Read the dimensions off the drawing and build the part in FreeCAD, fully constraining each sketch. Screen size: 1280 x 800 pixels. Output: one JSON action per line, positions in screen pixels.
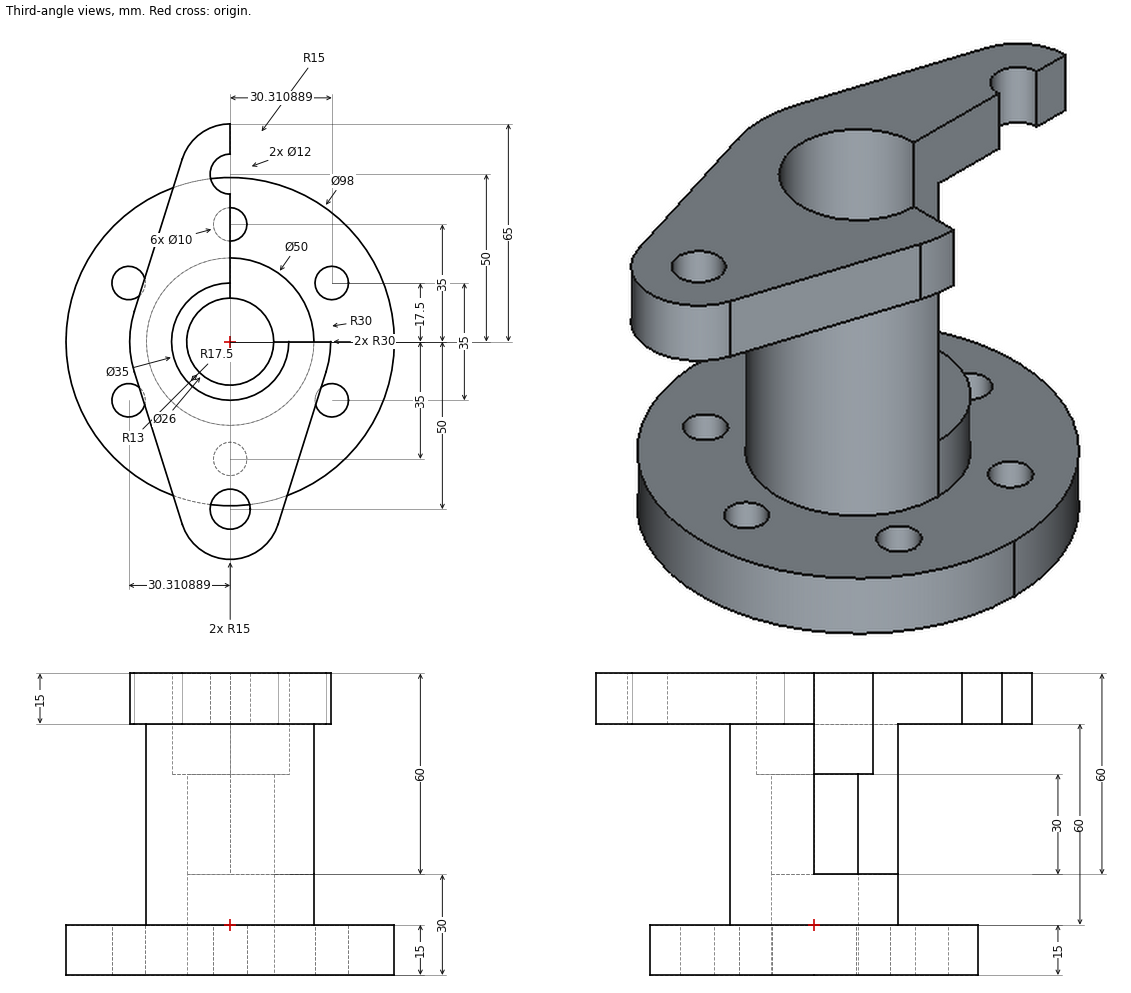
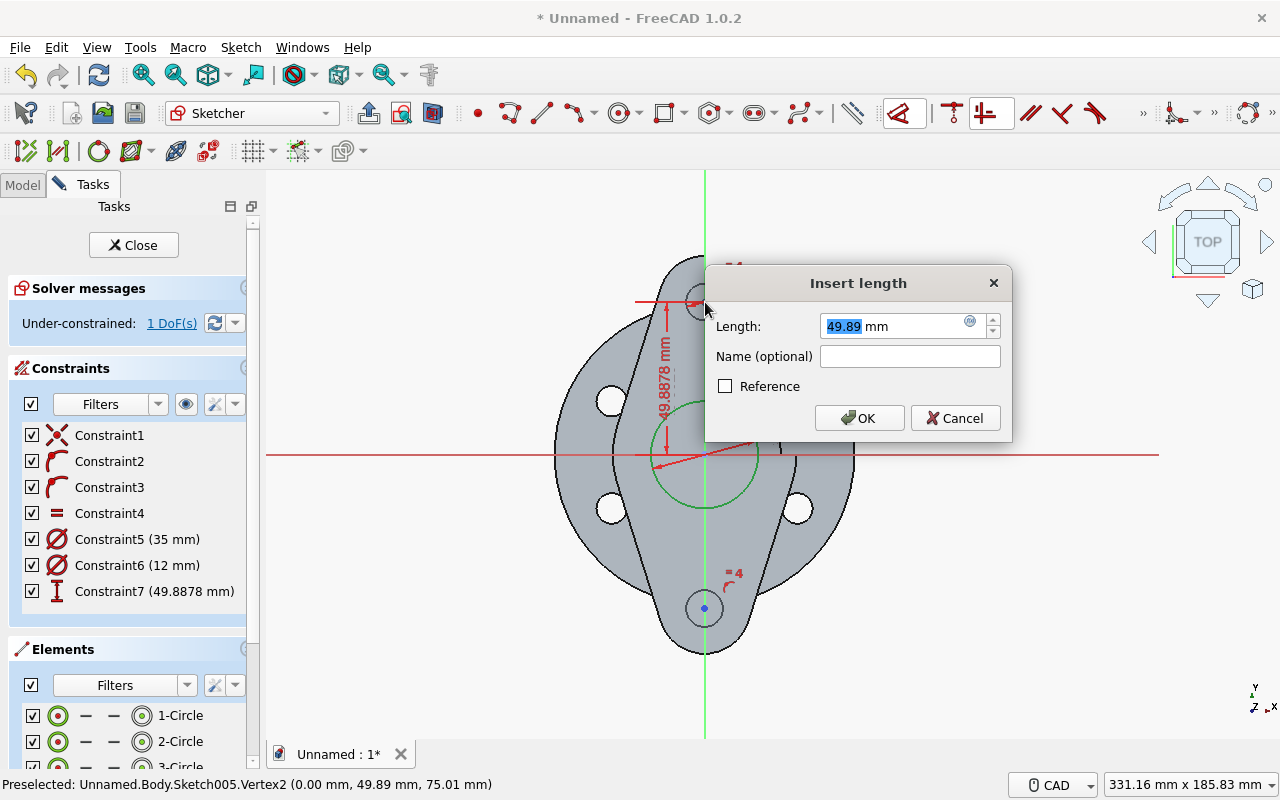
{"action": "type", "text": "50"}
{"action": "key", "text": "Return"}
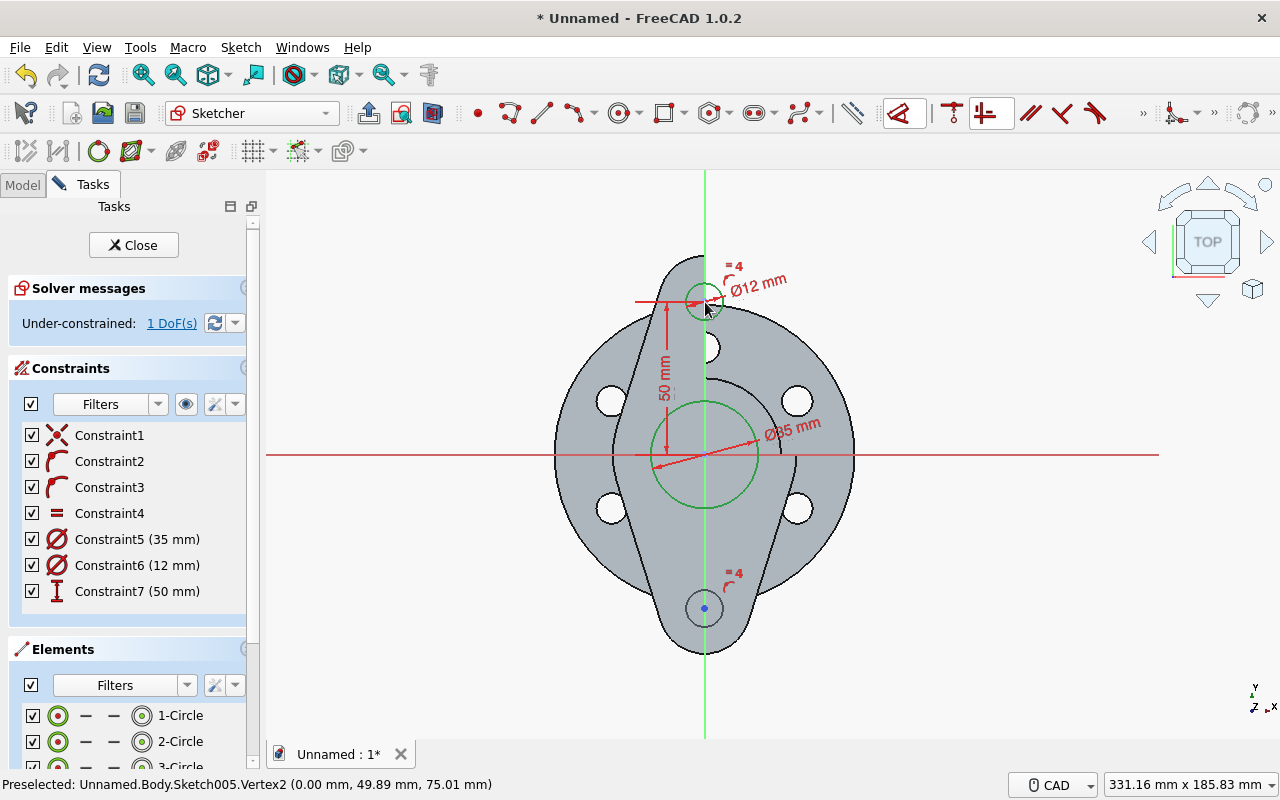
{"action": "left_click", "coordinate": [705, 609]}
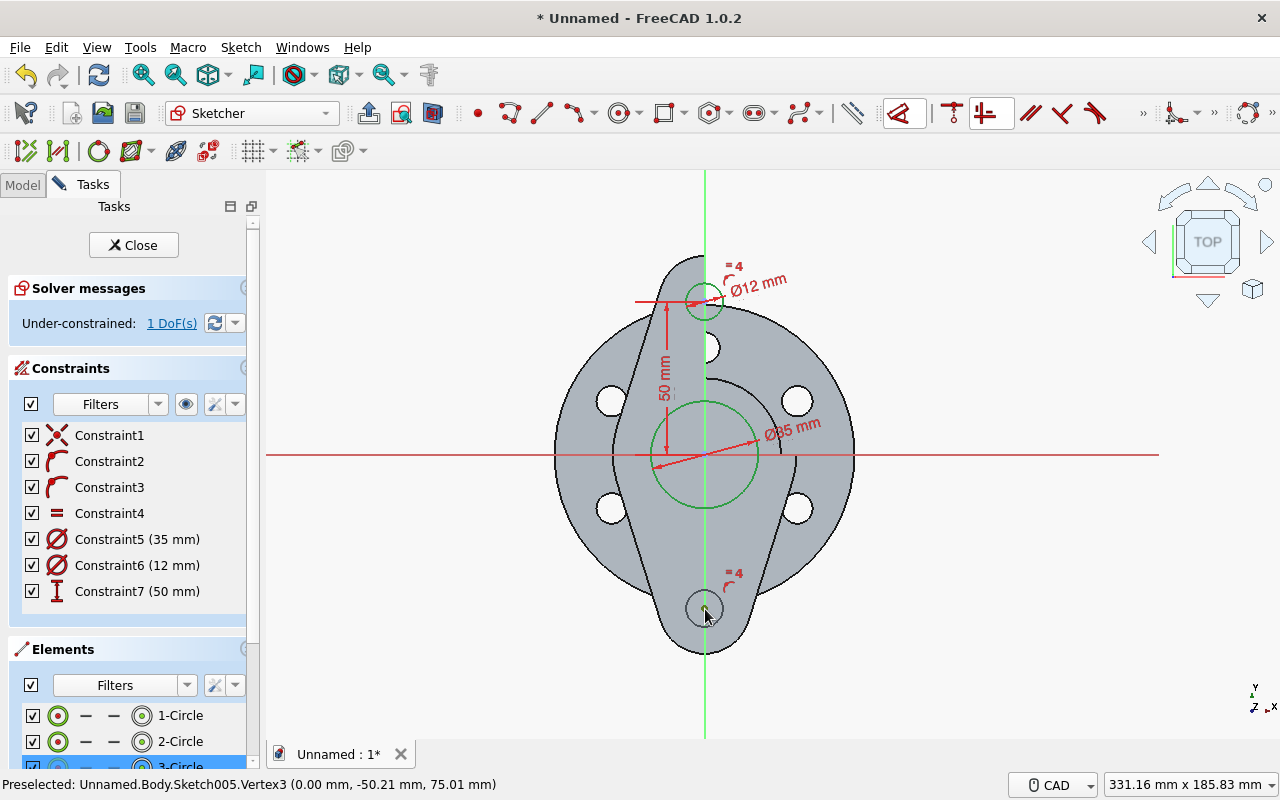
{"action": "key", "text": "i"}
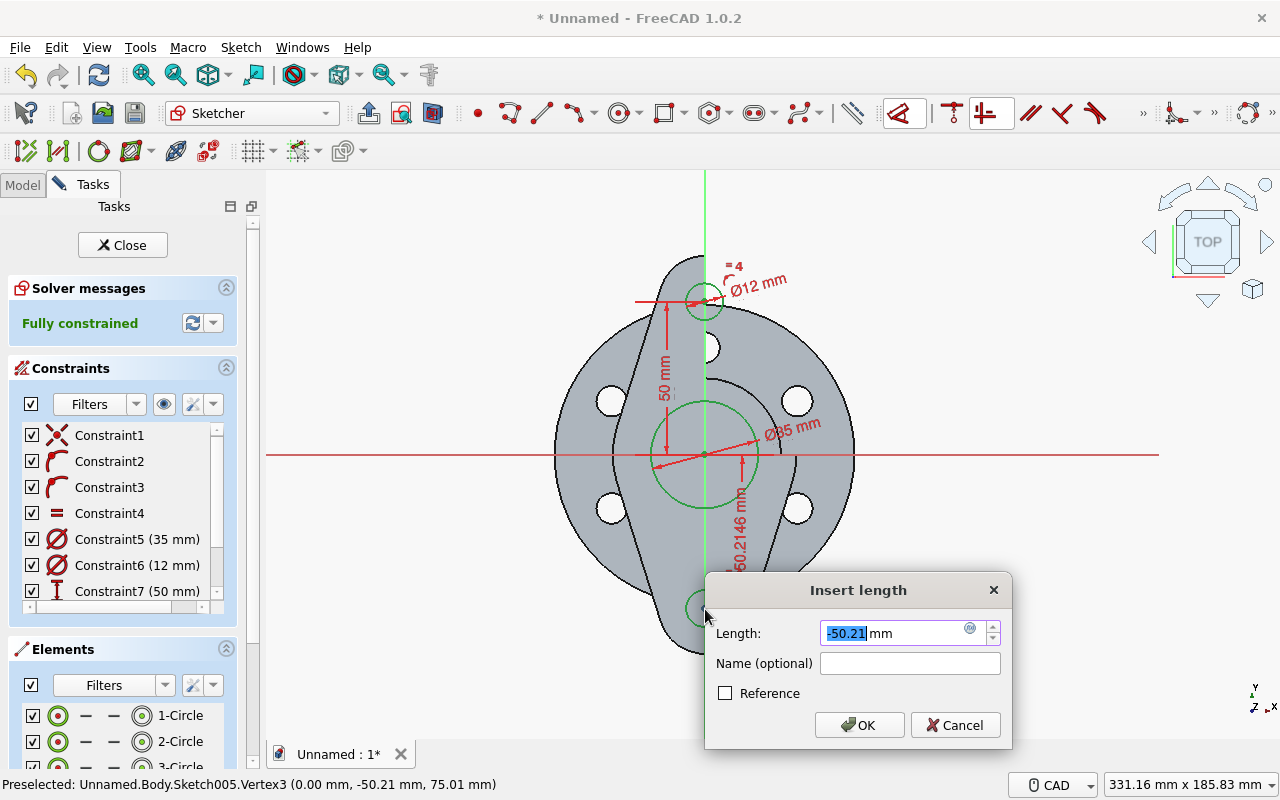
{"action": "type", "text": "-50"}
{"action": "key", "text": "Return"}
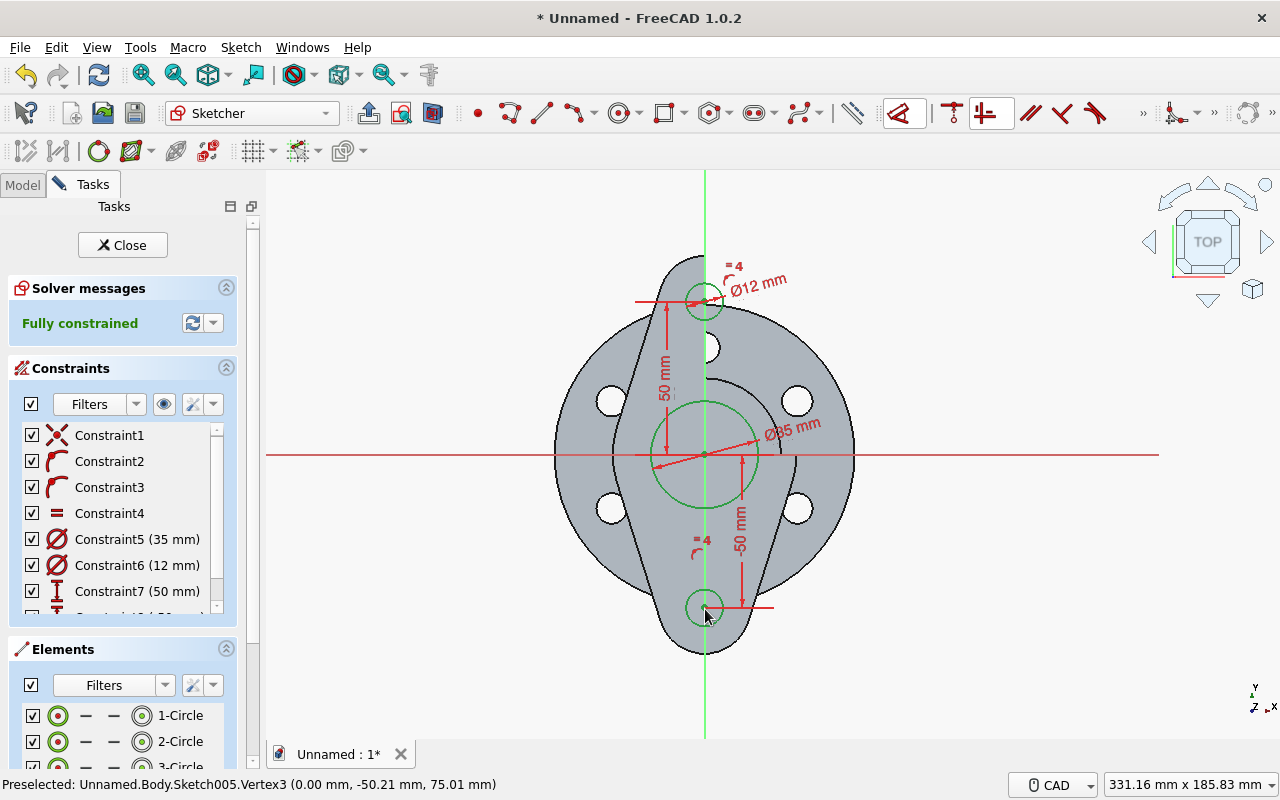
{"action": "left_click", "coordinate": [123, 245]}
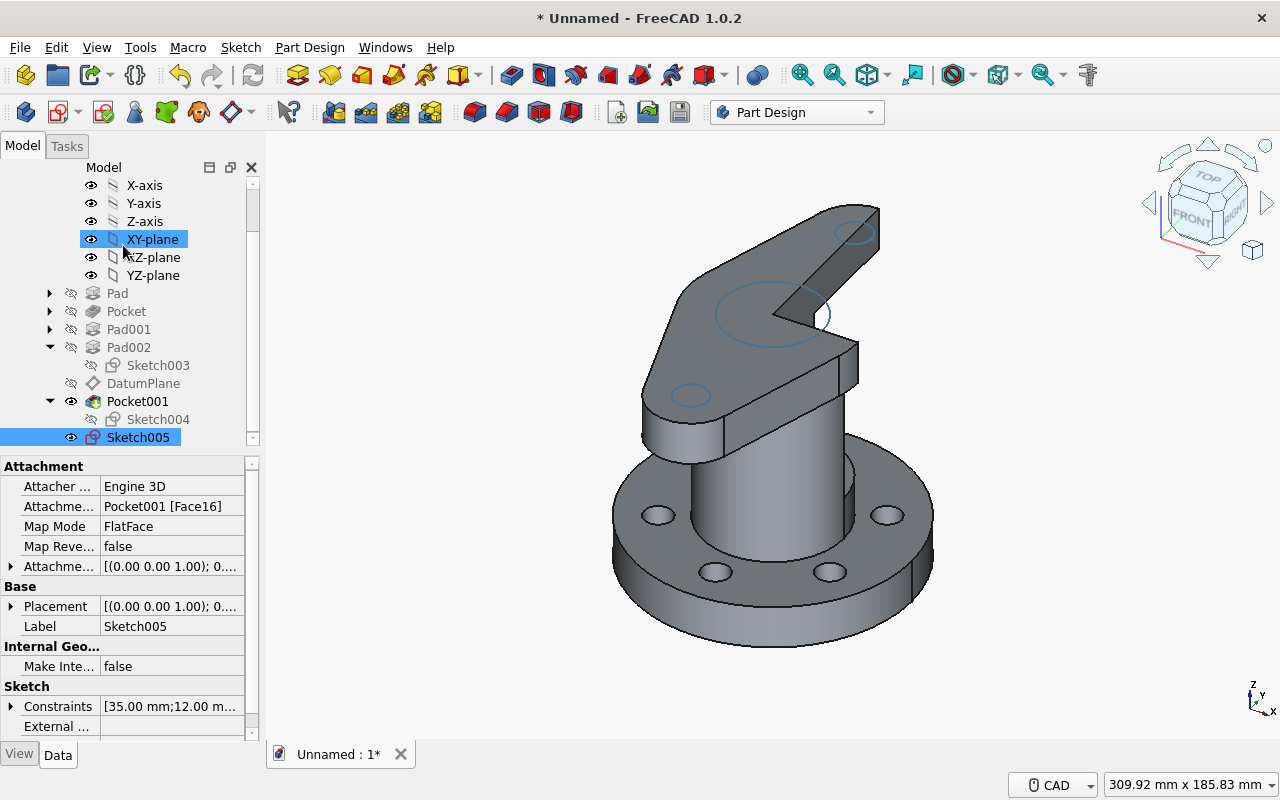
{"action": "left_click", "coordinate": [512, 76]}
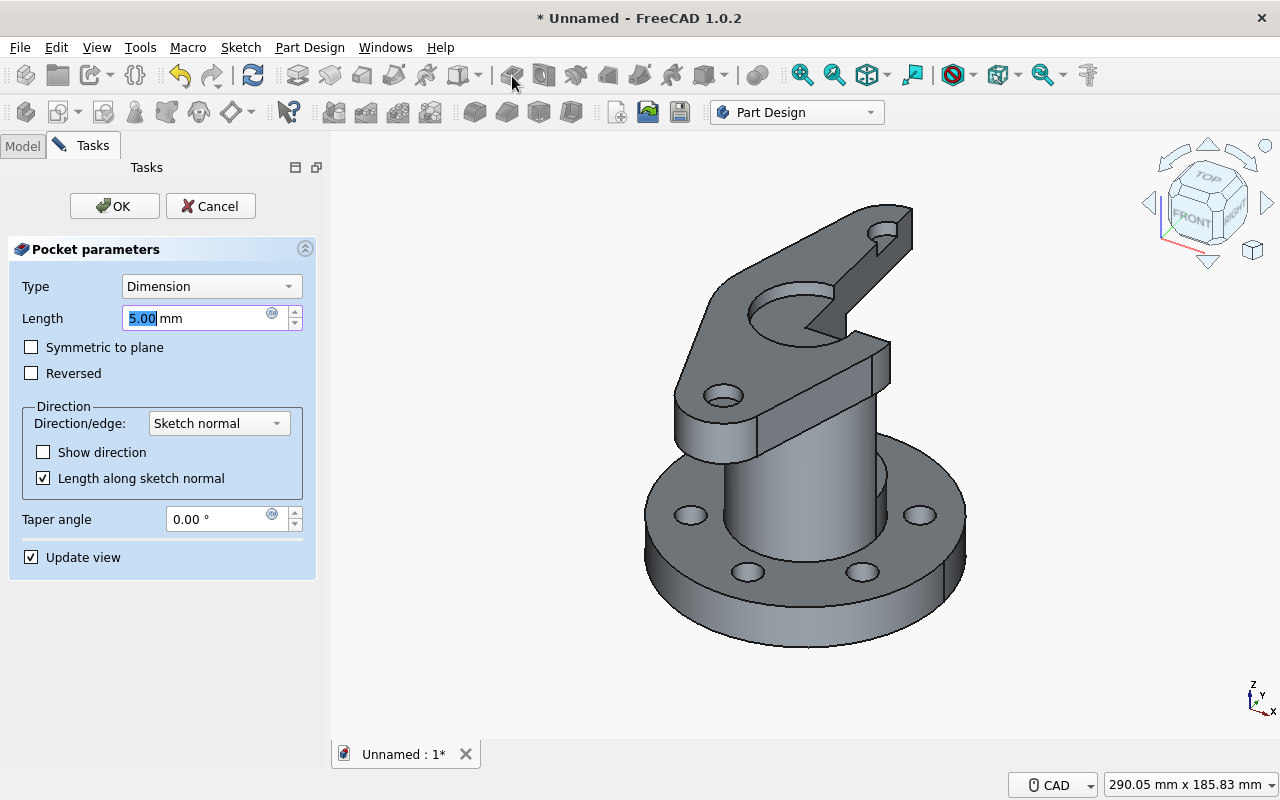
{"action": "type", "text": "60"}
{"action": "key", "text": "Tab"}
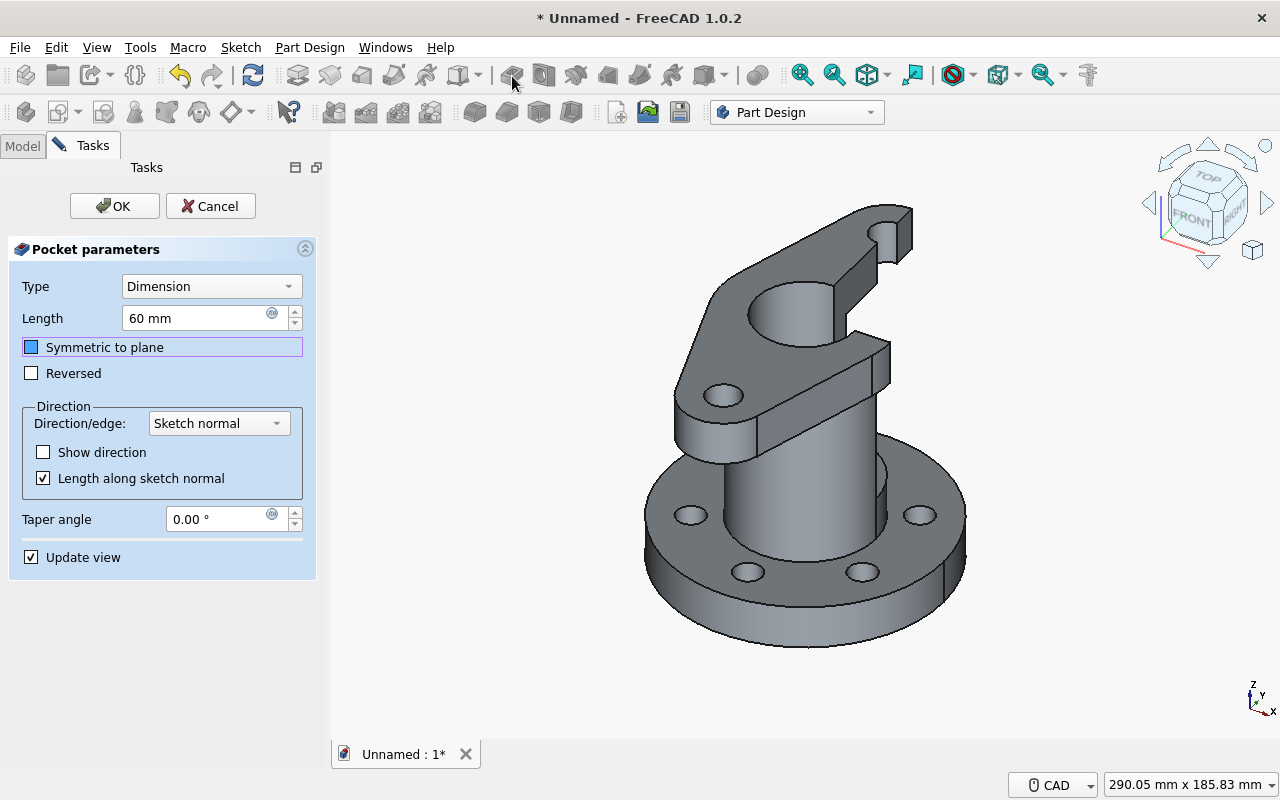
{"action": "left_click", "coordinate": [115, 206]}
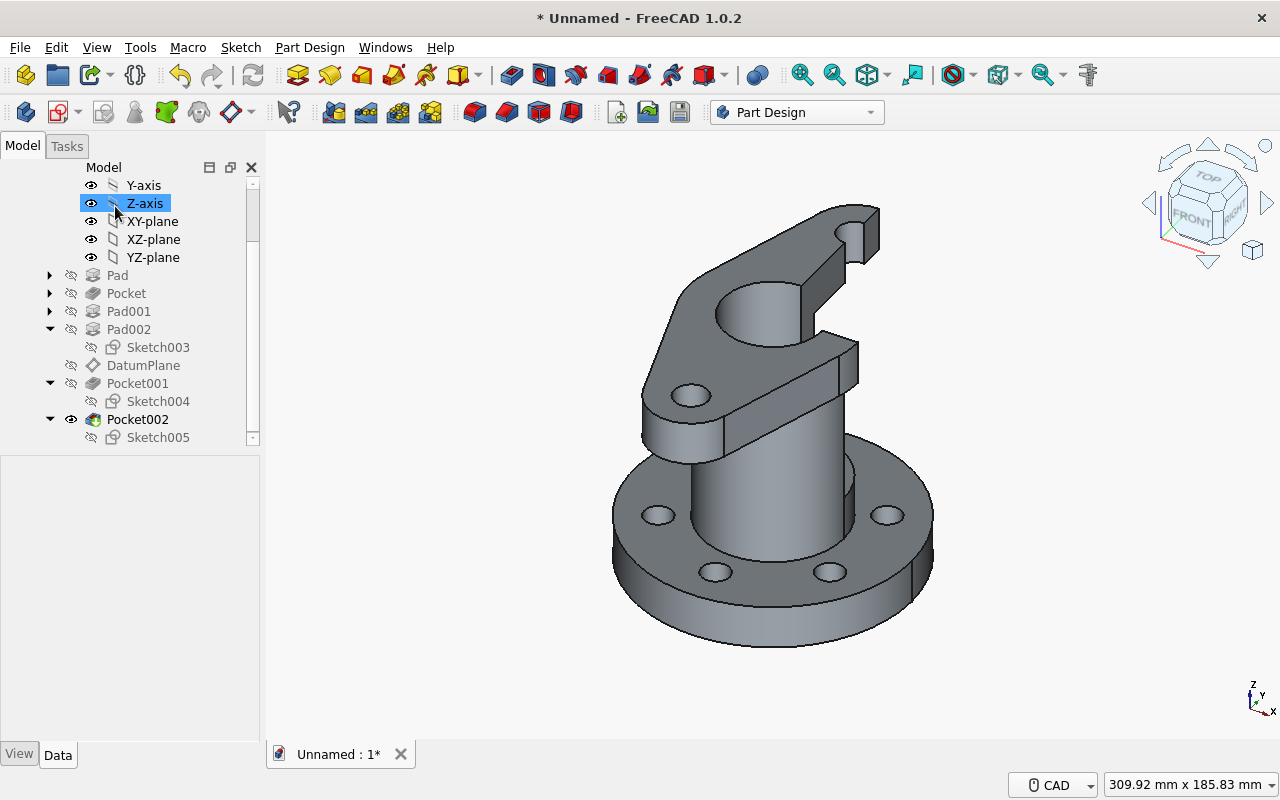
{"action": "scroll", "coordinate": [160, 307], "scroll_direction": "down", "scroll_amount": 3}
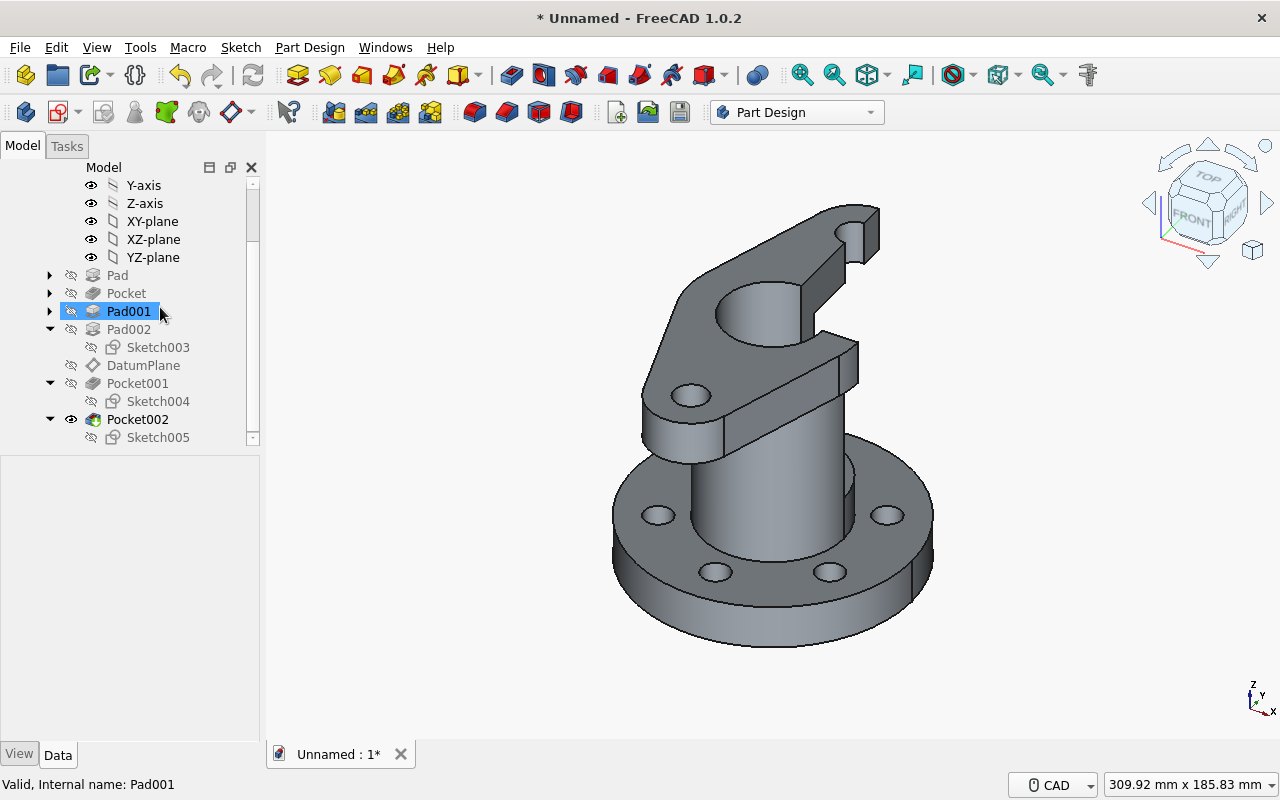
{"action": "scroll", "coordinate": [160, 307], "scroll_direction": "up", "scroll_amount": 15}